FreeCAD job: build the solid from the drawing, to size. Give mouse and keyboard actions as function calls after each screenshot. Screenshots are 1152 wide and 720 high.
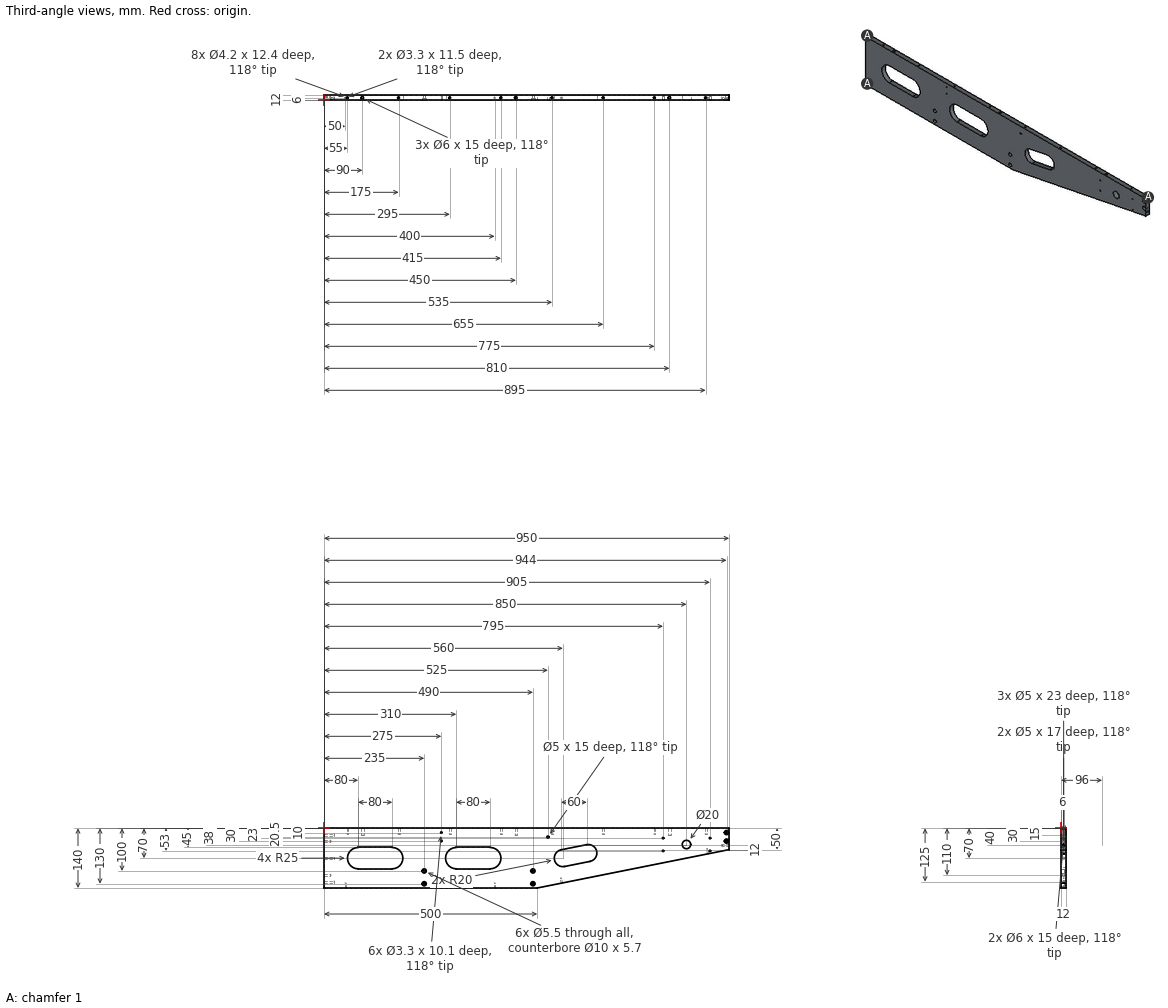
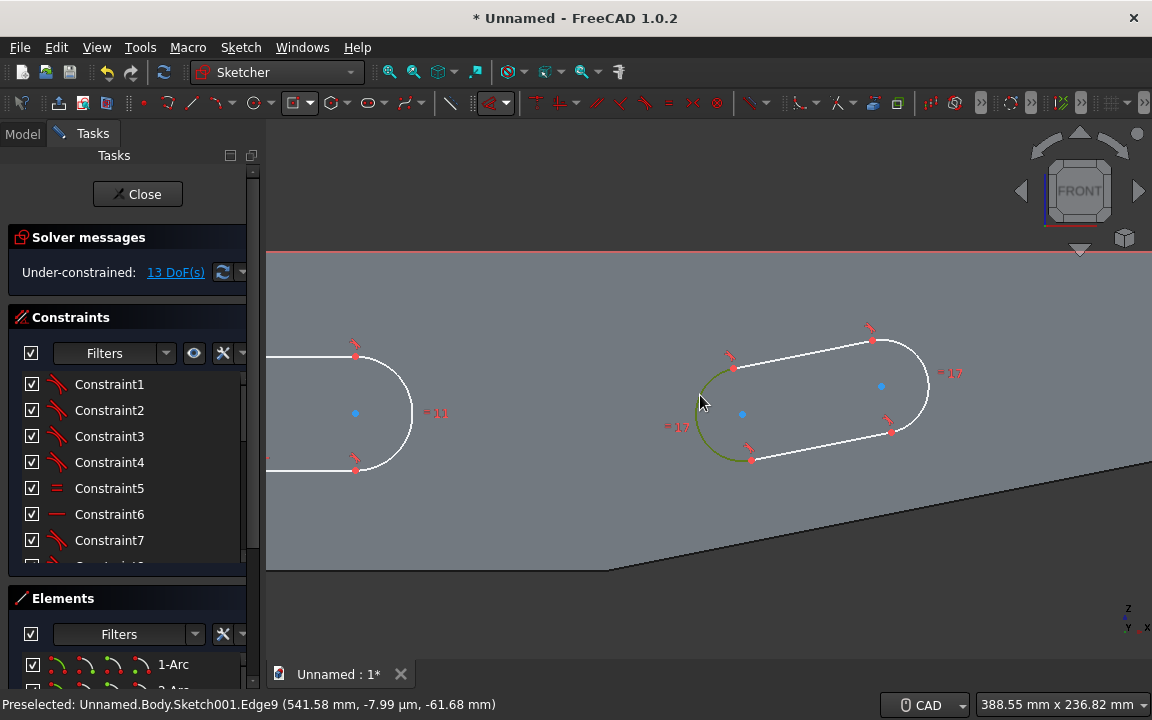
click(508, 104)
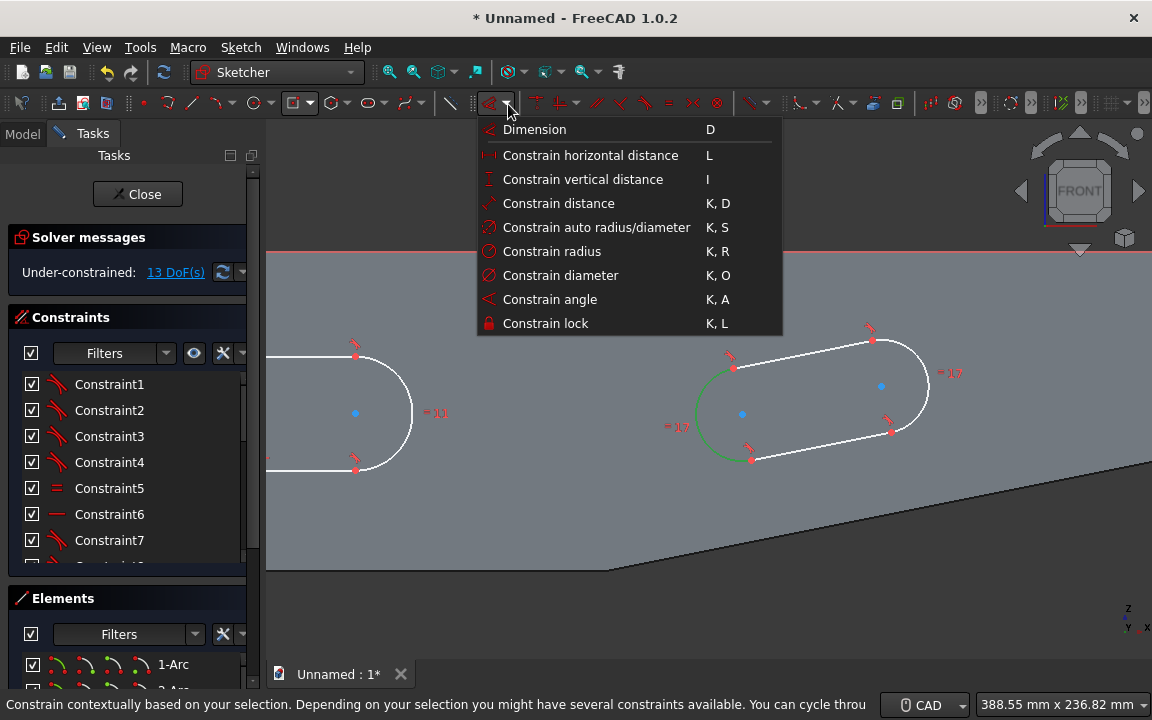
click(630, 251)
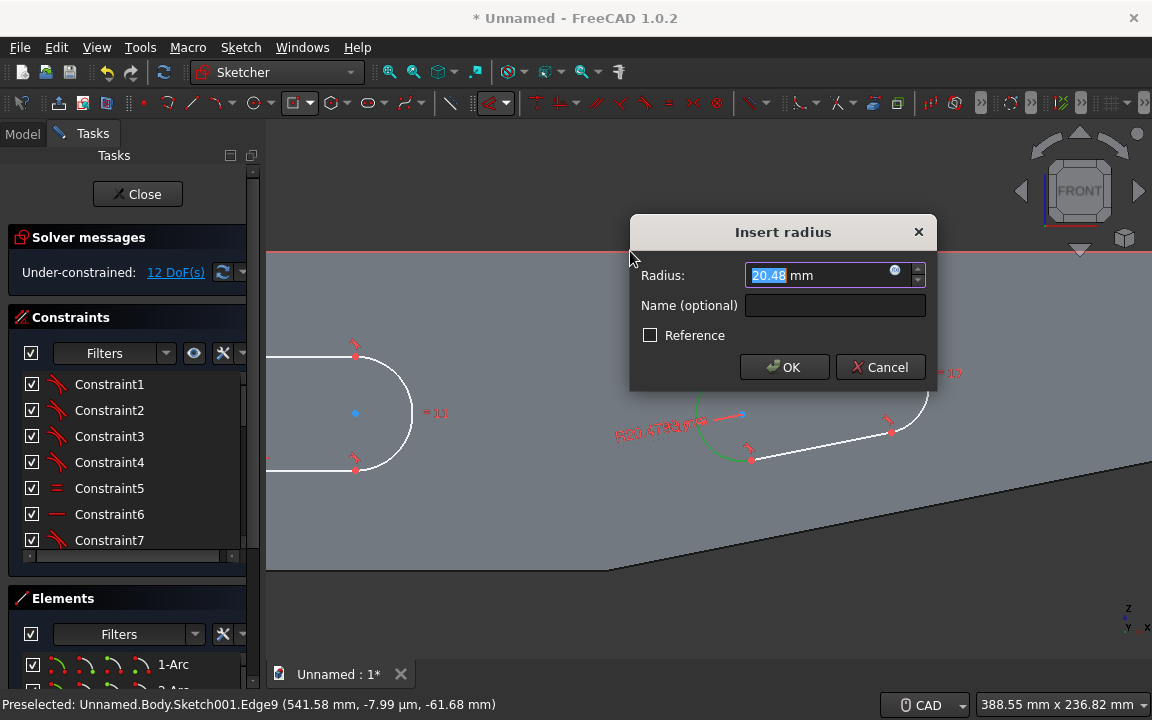
text(20)
key(Return)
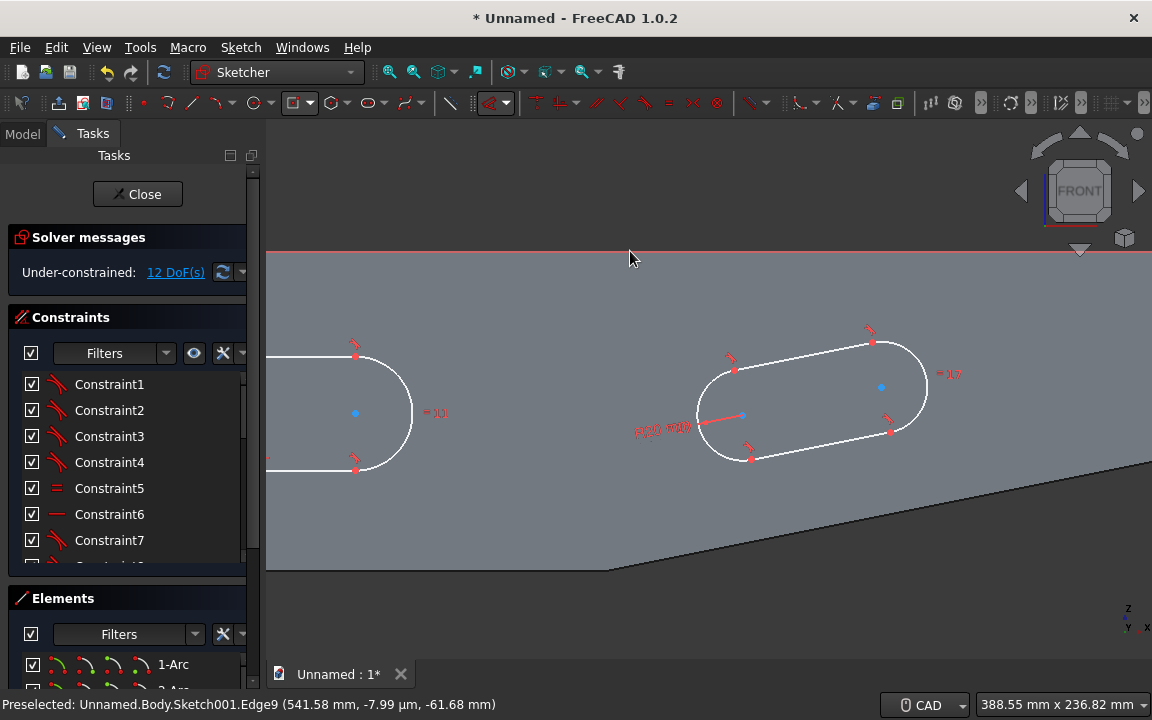
scroll(704, 398, down, 7)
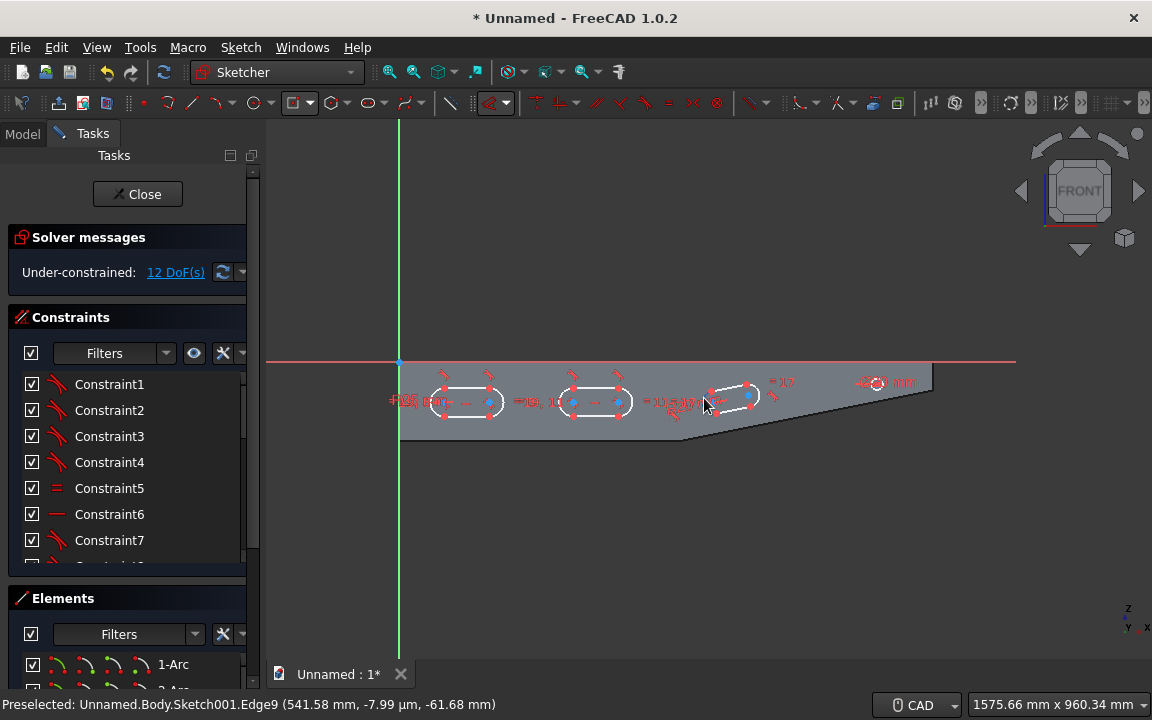
click(458, 388)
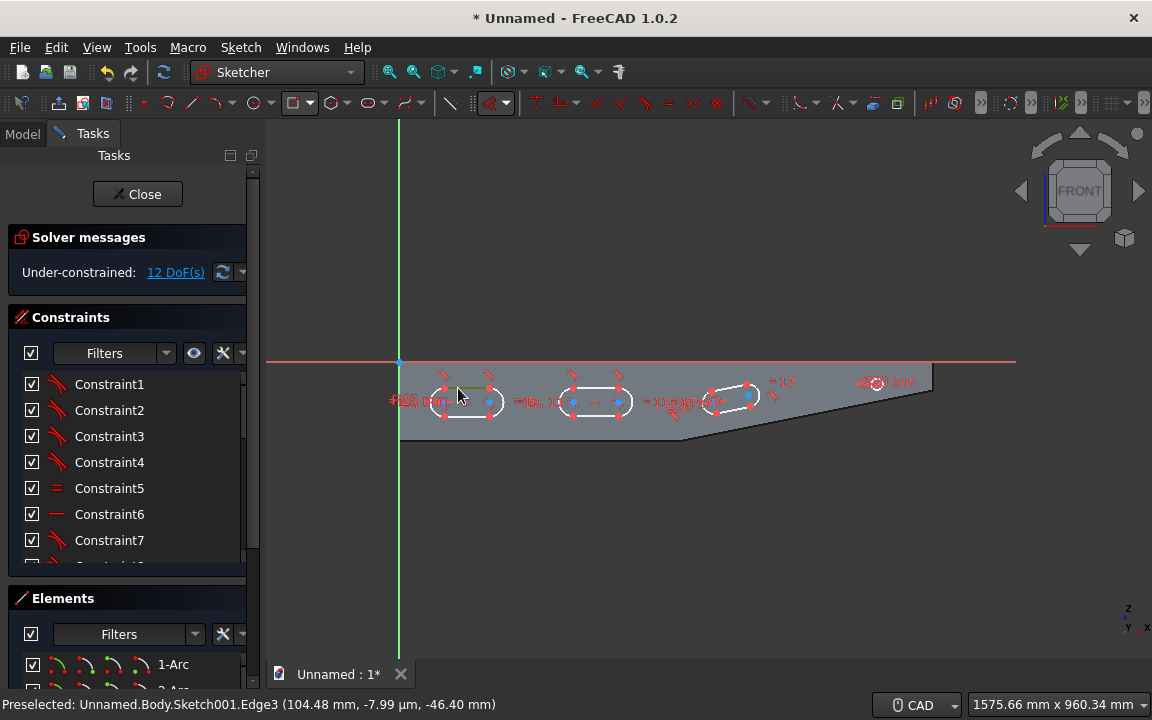
key(l)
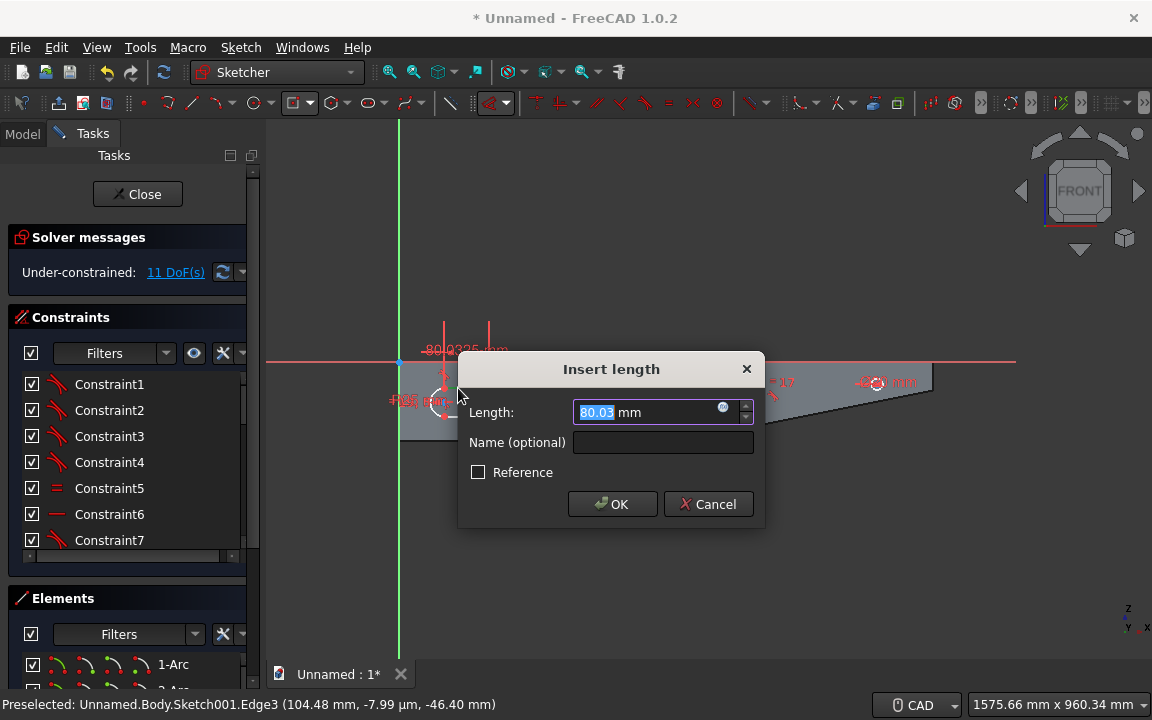
text(80)
key(Return)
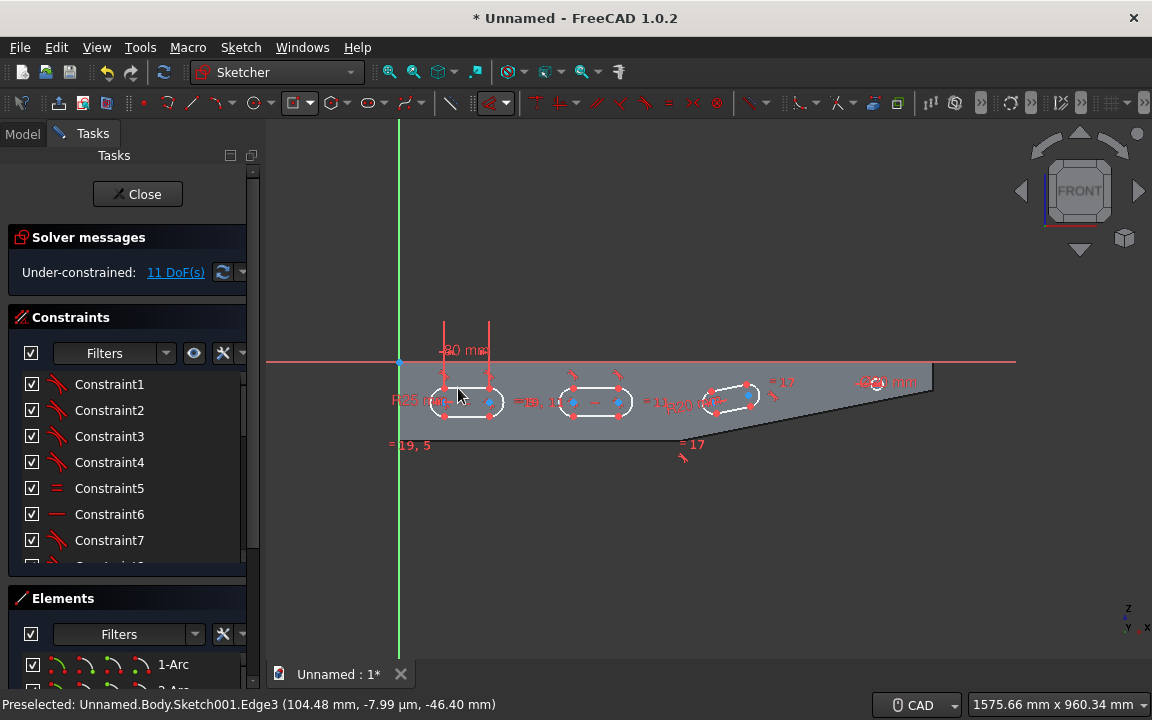
click(587, 388)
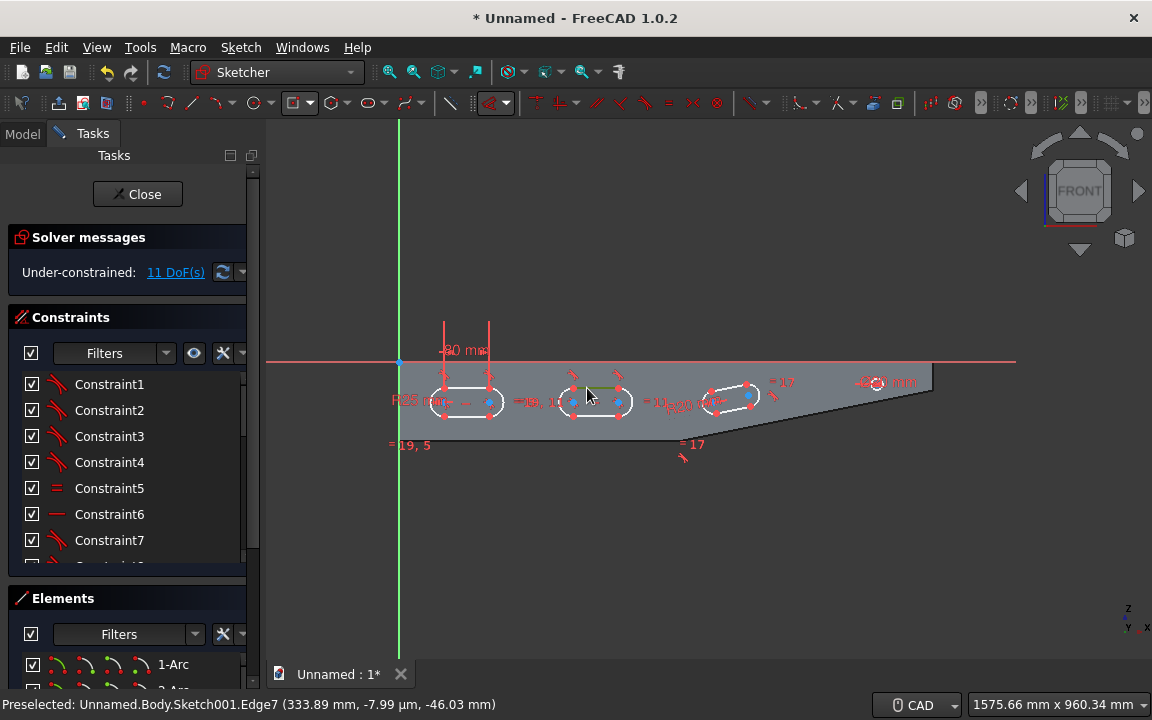
key(l)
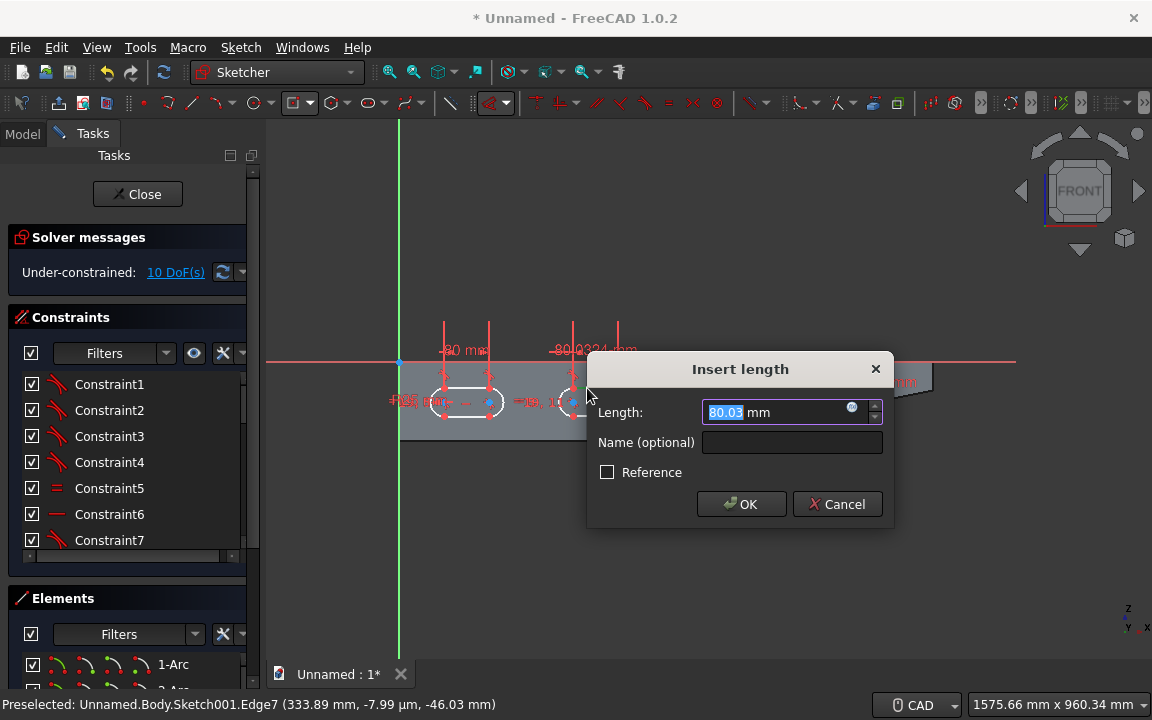
text(80)
key(Return)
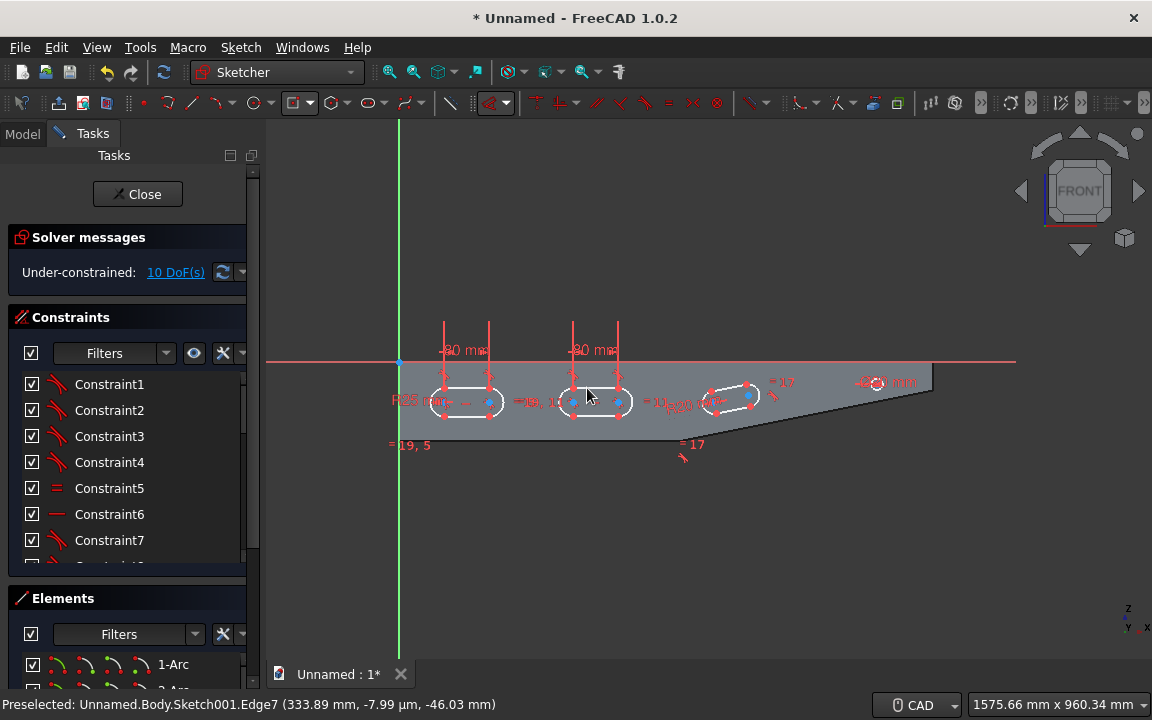
scroll(877, 384, up, 4)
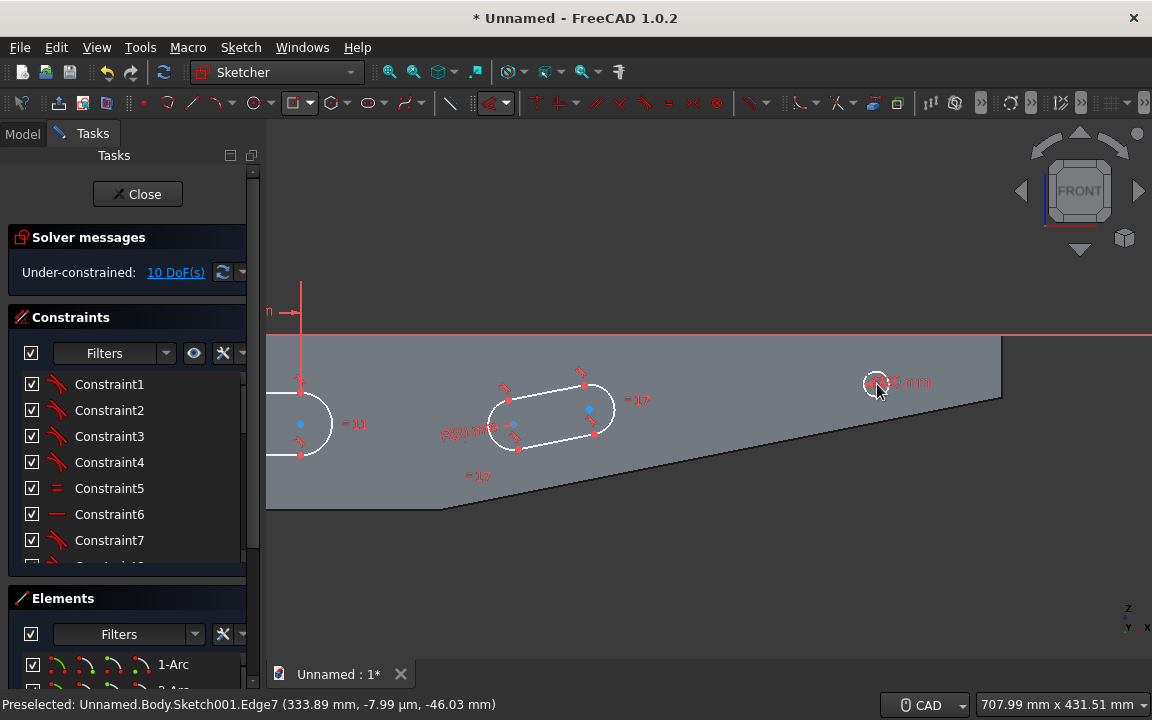
click(876, 384)